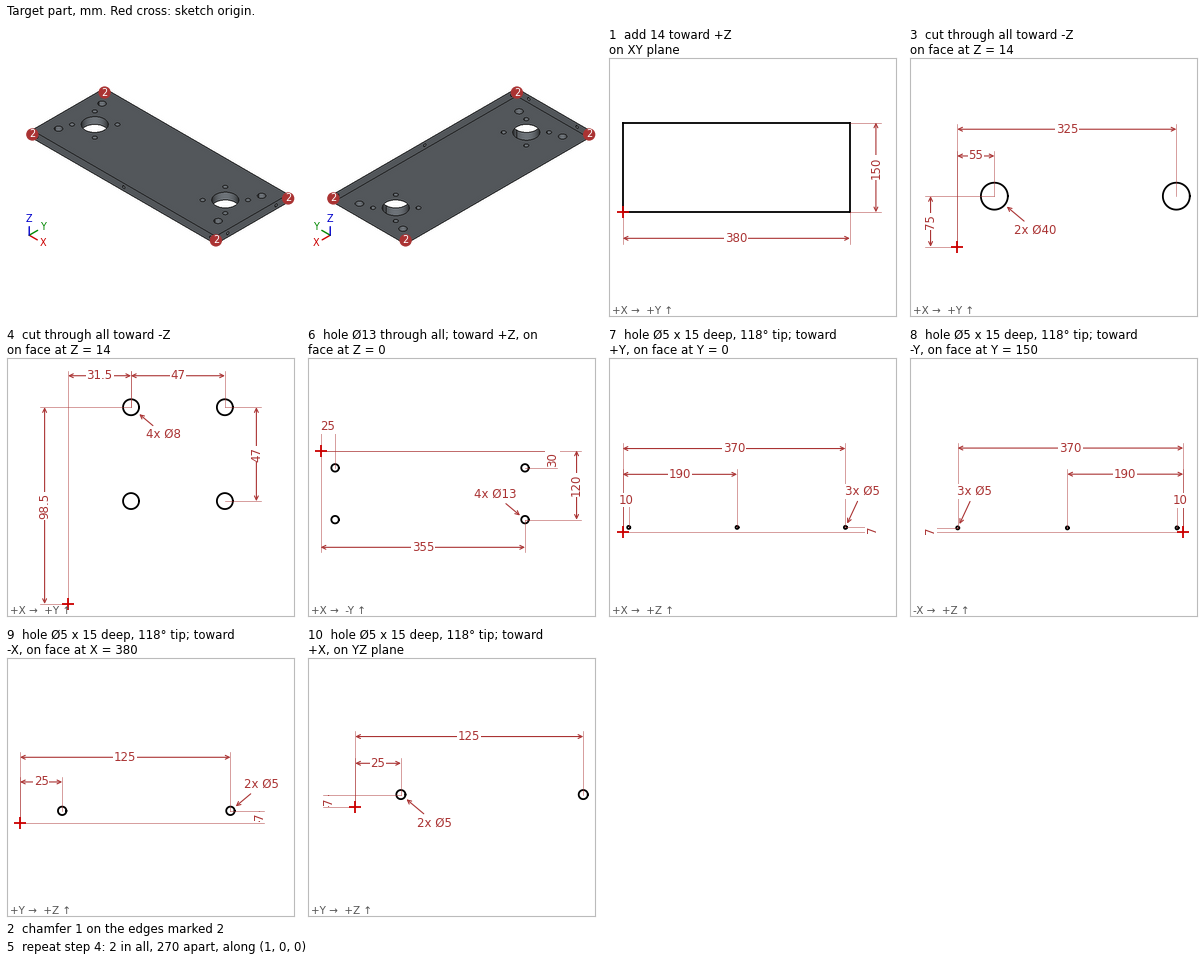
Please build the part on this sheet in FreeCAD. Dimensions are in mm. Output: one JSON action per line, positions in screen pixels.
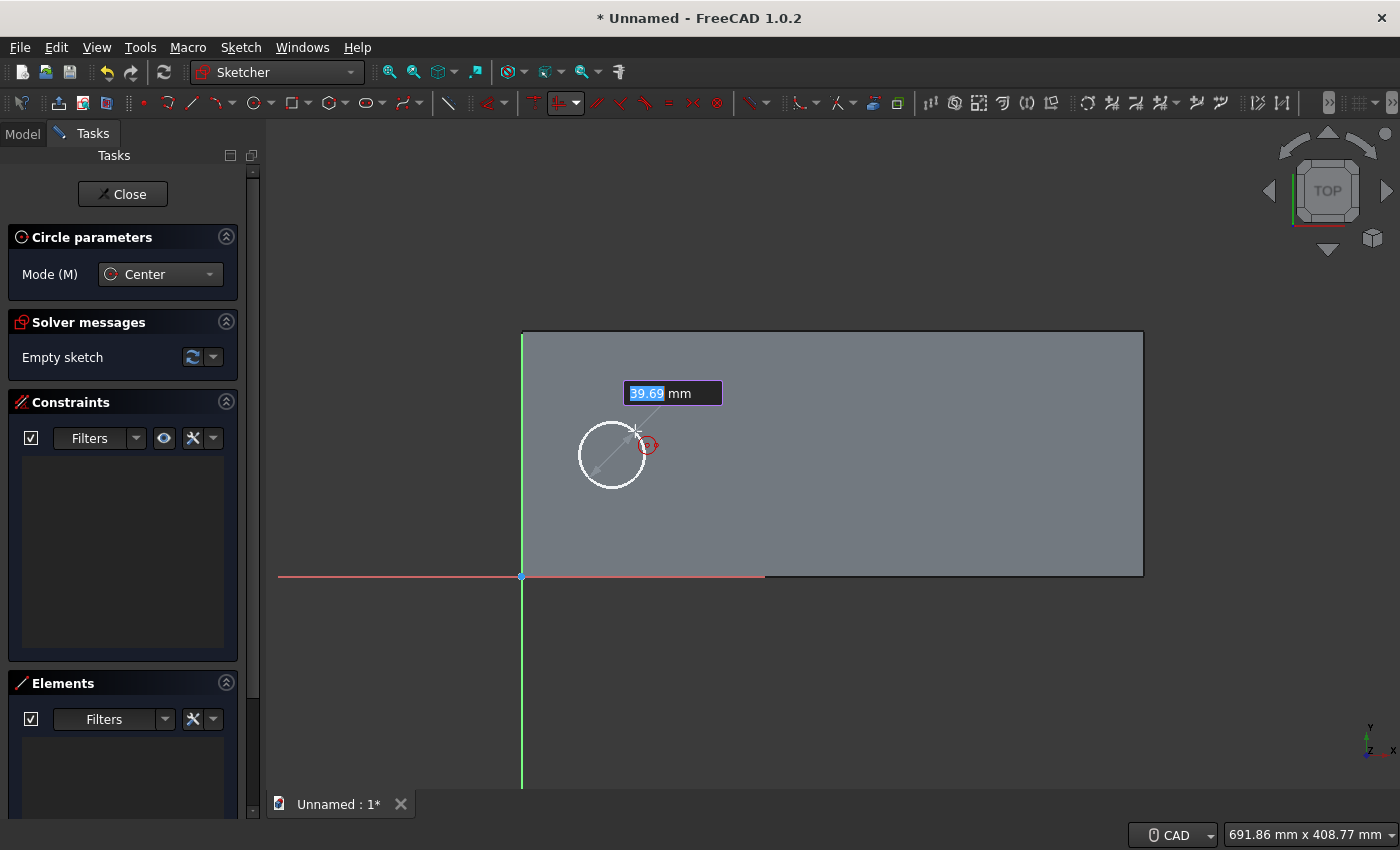
{"action": "type", "text": "40"}
{"action": "key", "text": "Return"}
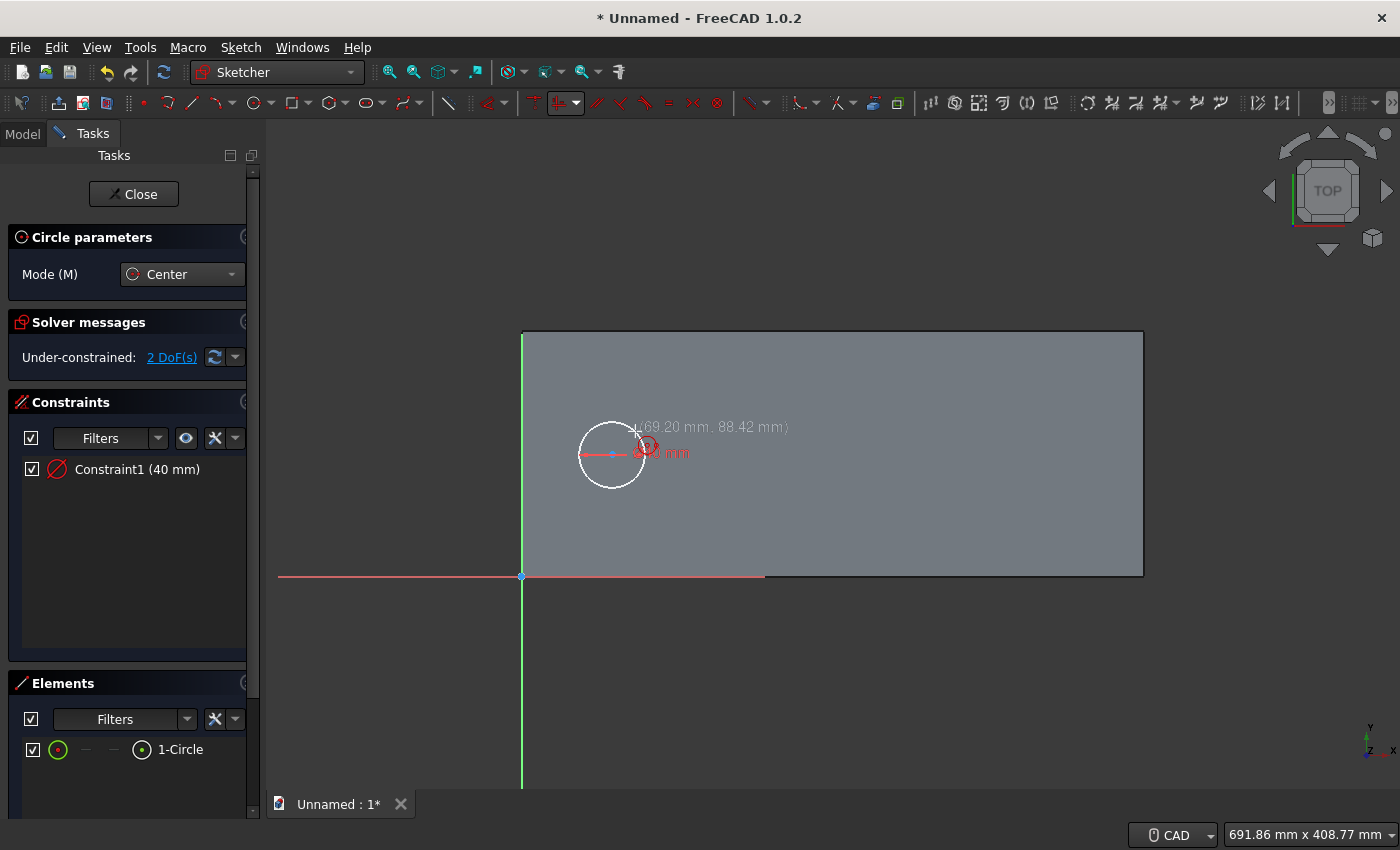
{"action": "left_click", "coordinate": [1054, 454]}
{"action": "mouse_move", "coordinate": [1077, 431]}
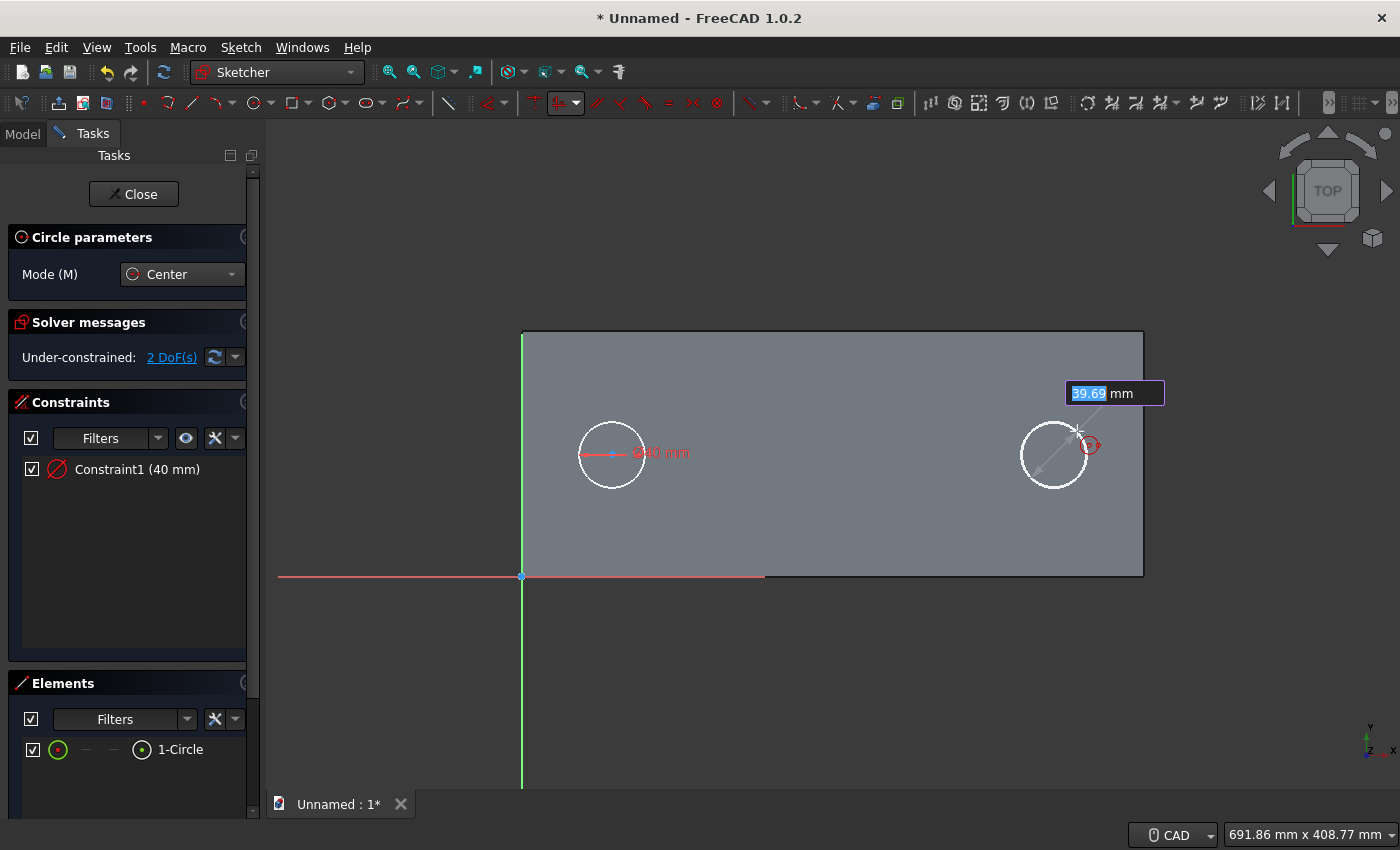
{"action": "type", "text": "40"}
{"action": "key", "text": "Return"}
{"action": "key", "text": "Escape"}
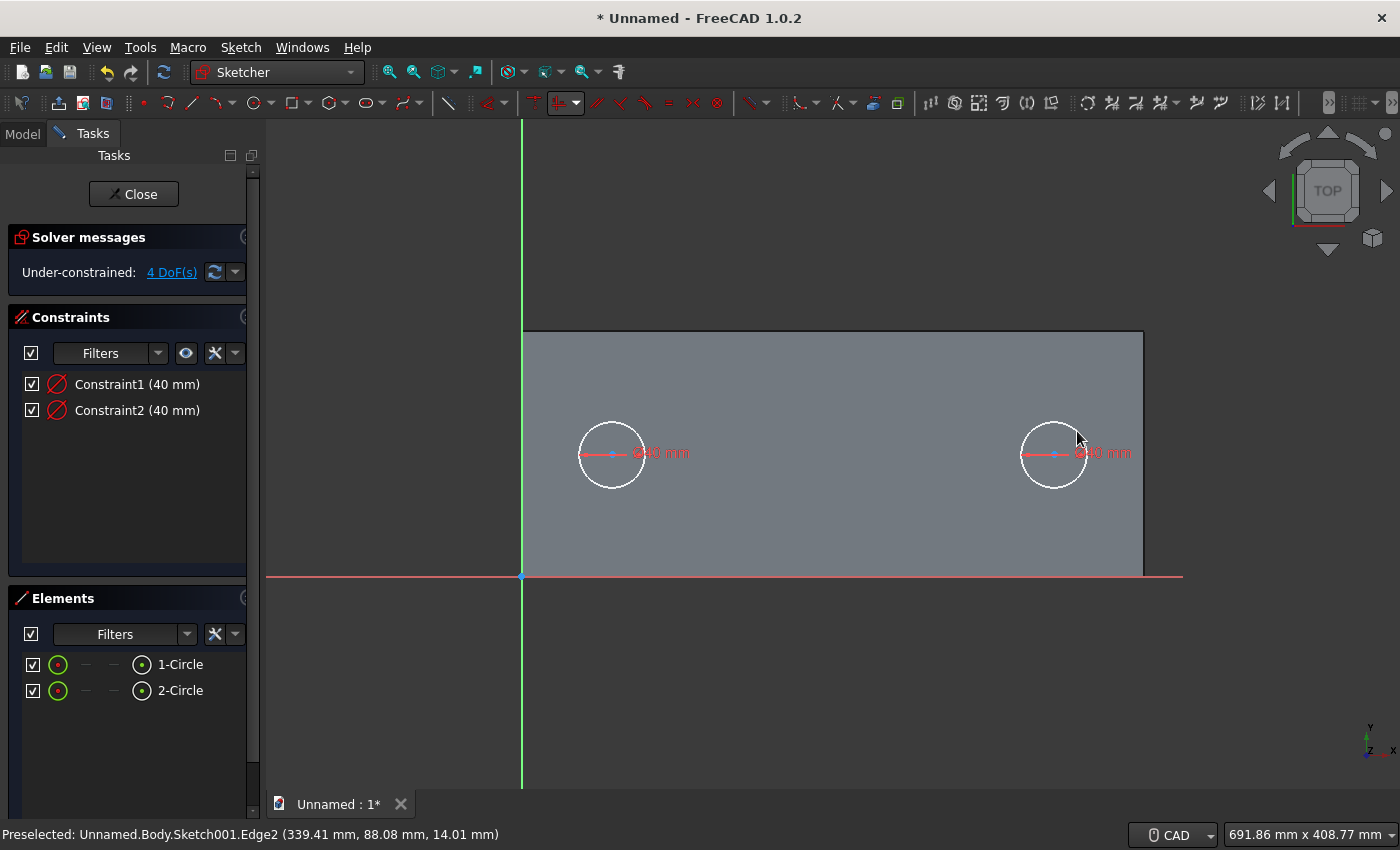
{"action": "left_click", "coordinate": [612, 455]}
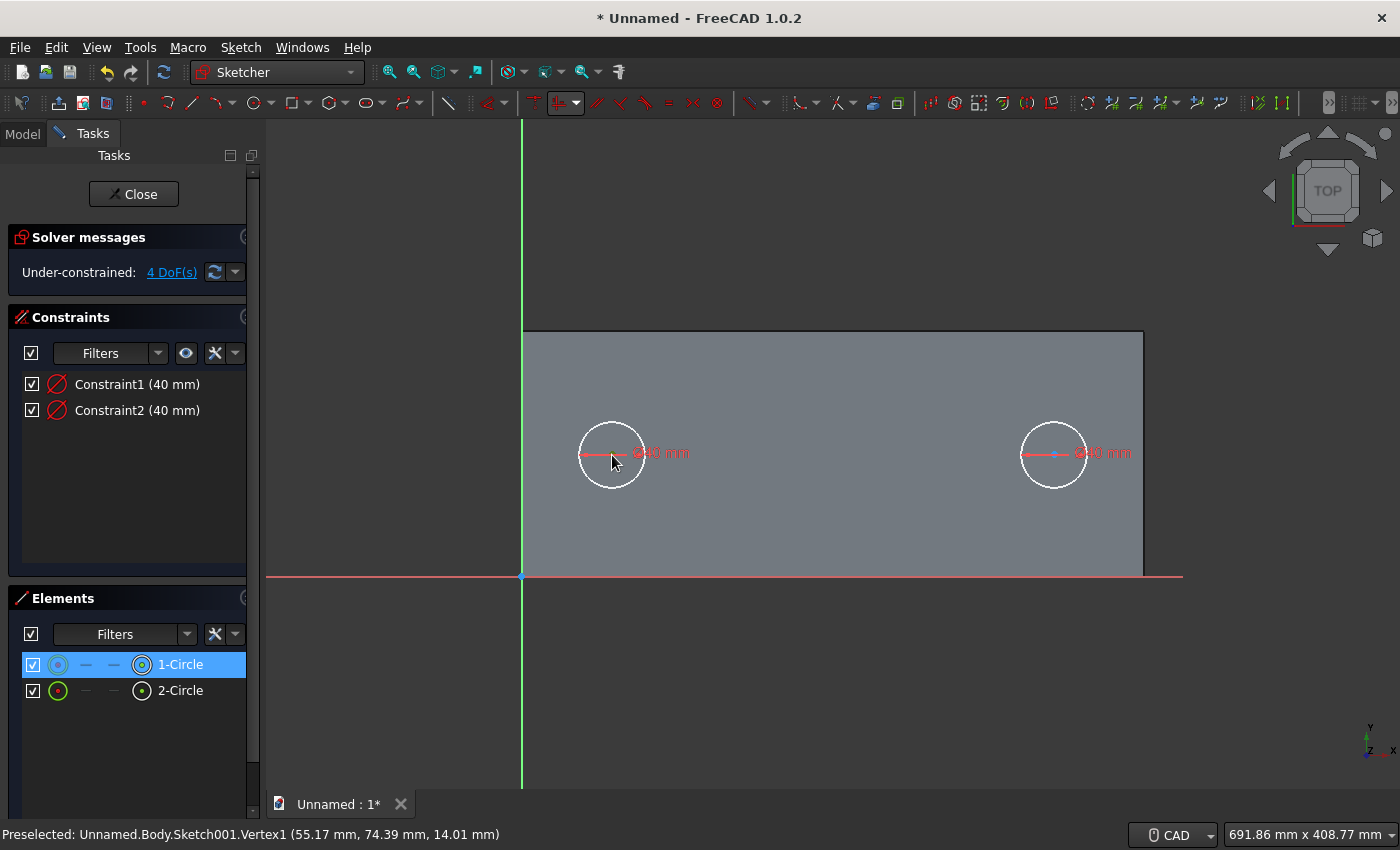
{"action": "left_click", "coordinate": [1054, 455]}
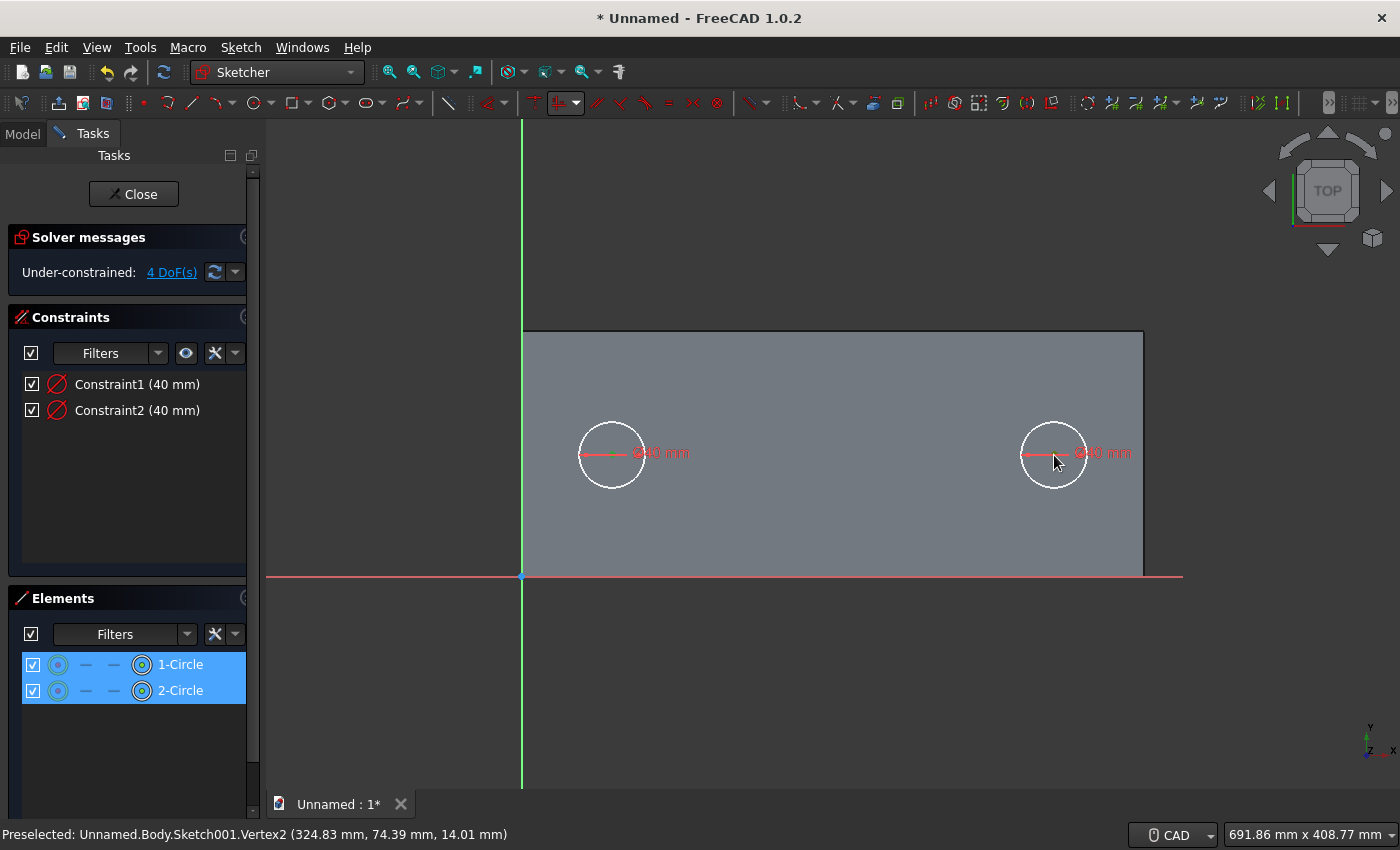
{"action": "key", "text": "h"}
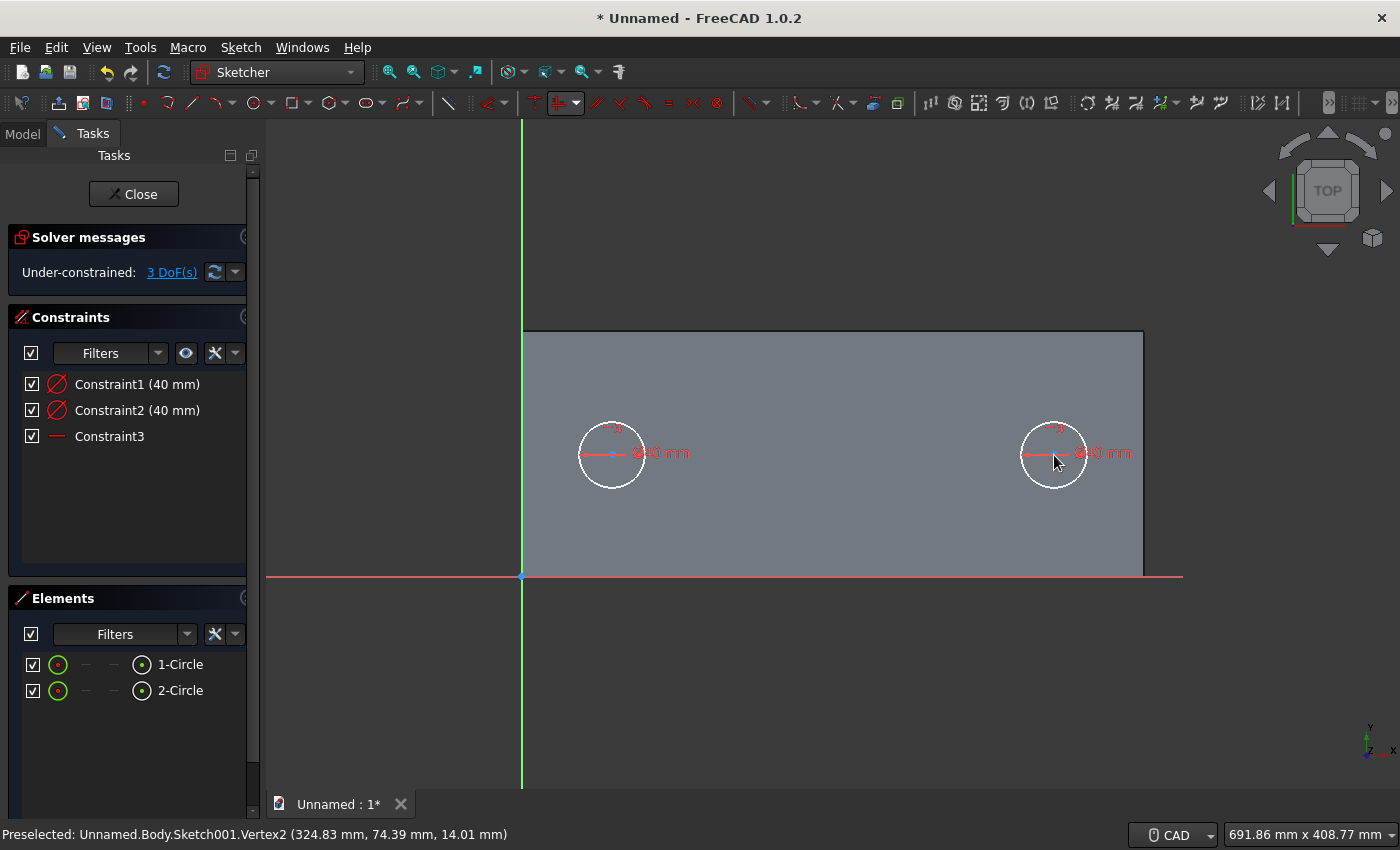
{"action": "key", "text": "d"}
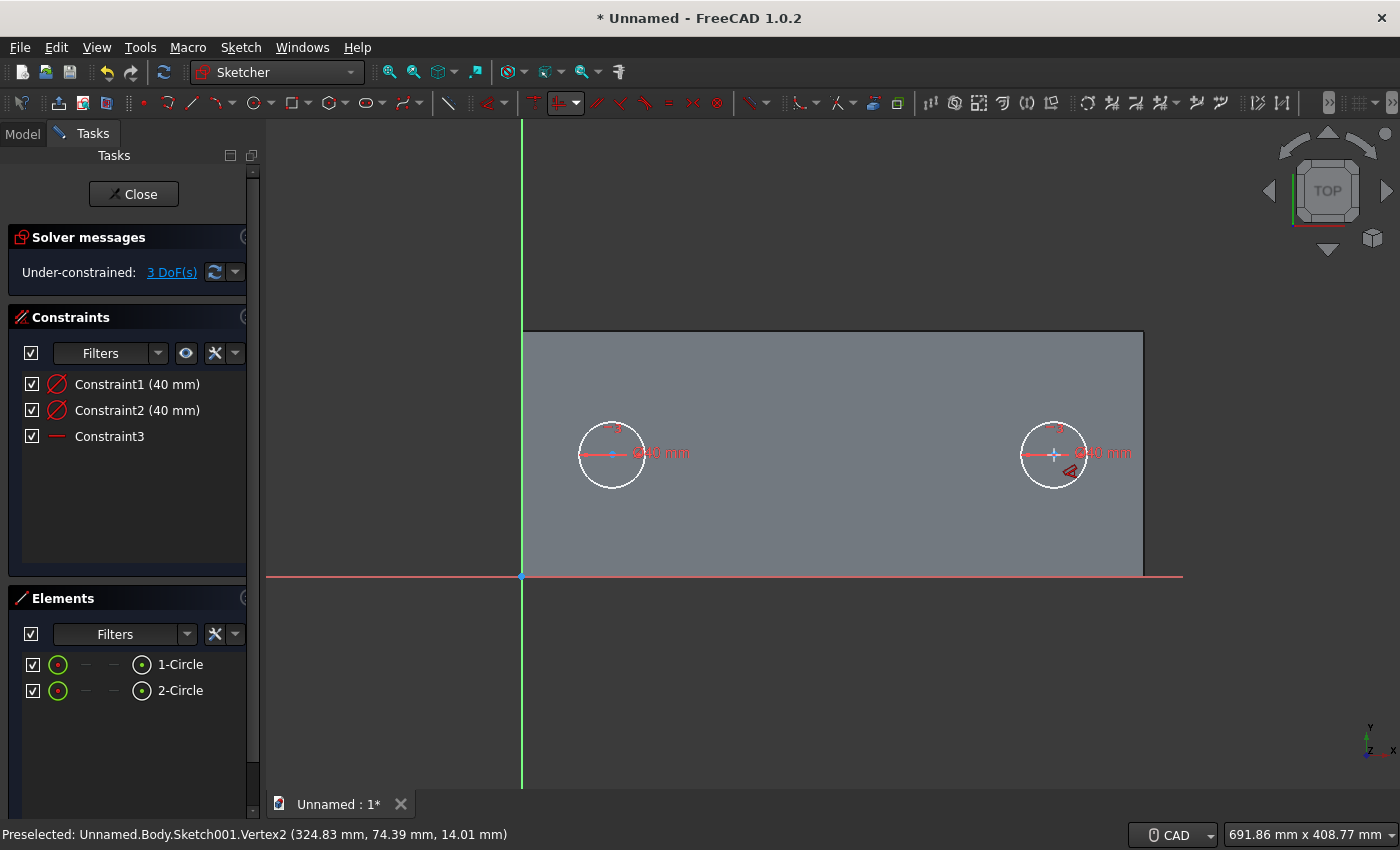
{"action": "left_click", "coordinate": [612, 455]}
{"action": "left_click", "coordinate": [567, 611]}